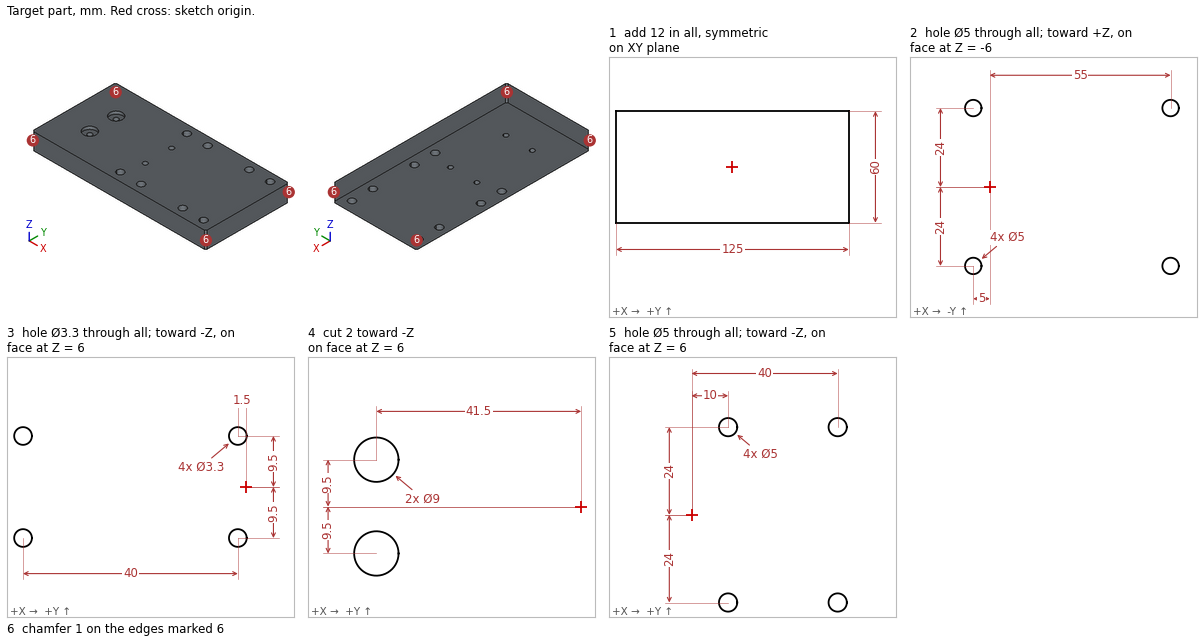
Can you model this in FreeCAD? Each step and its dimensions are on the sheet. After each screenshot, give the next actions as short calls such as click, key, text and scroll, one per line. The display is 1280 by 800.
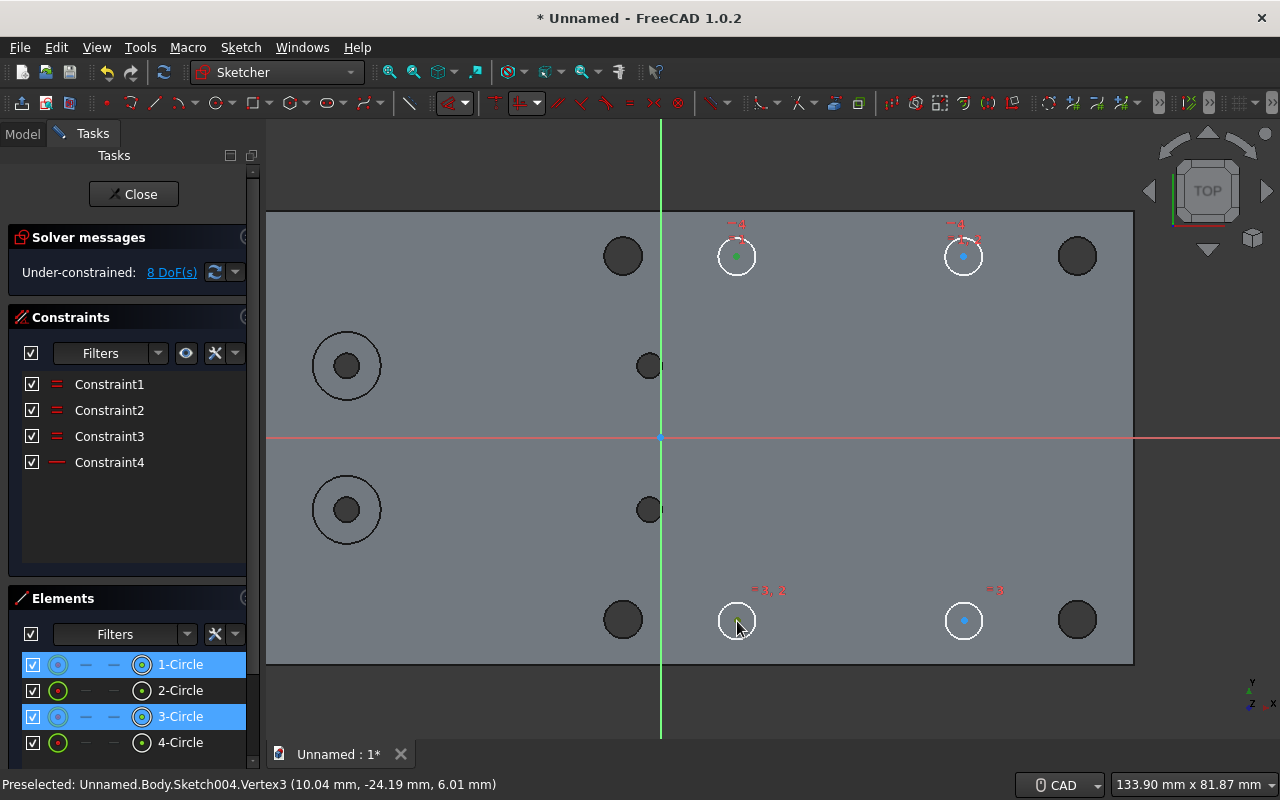
key(v)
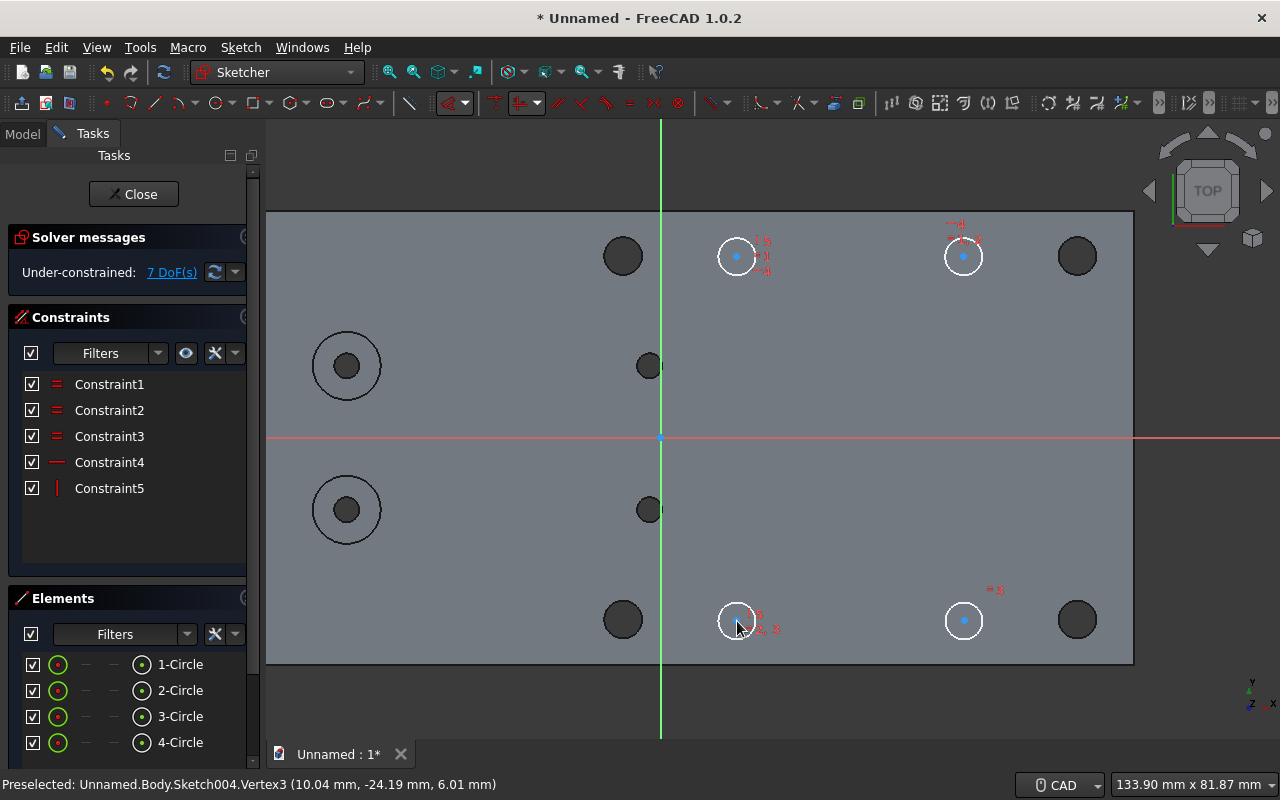
click(964, 257)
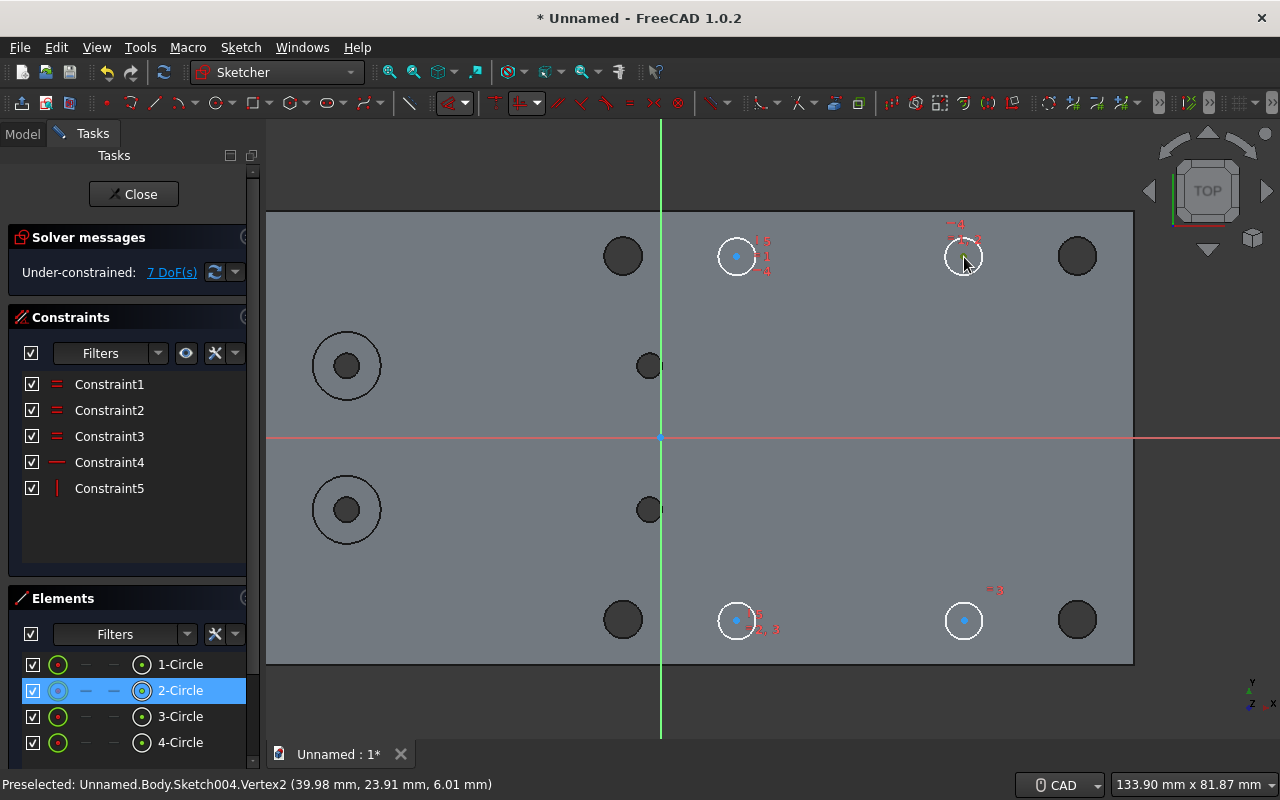
click(964, 621)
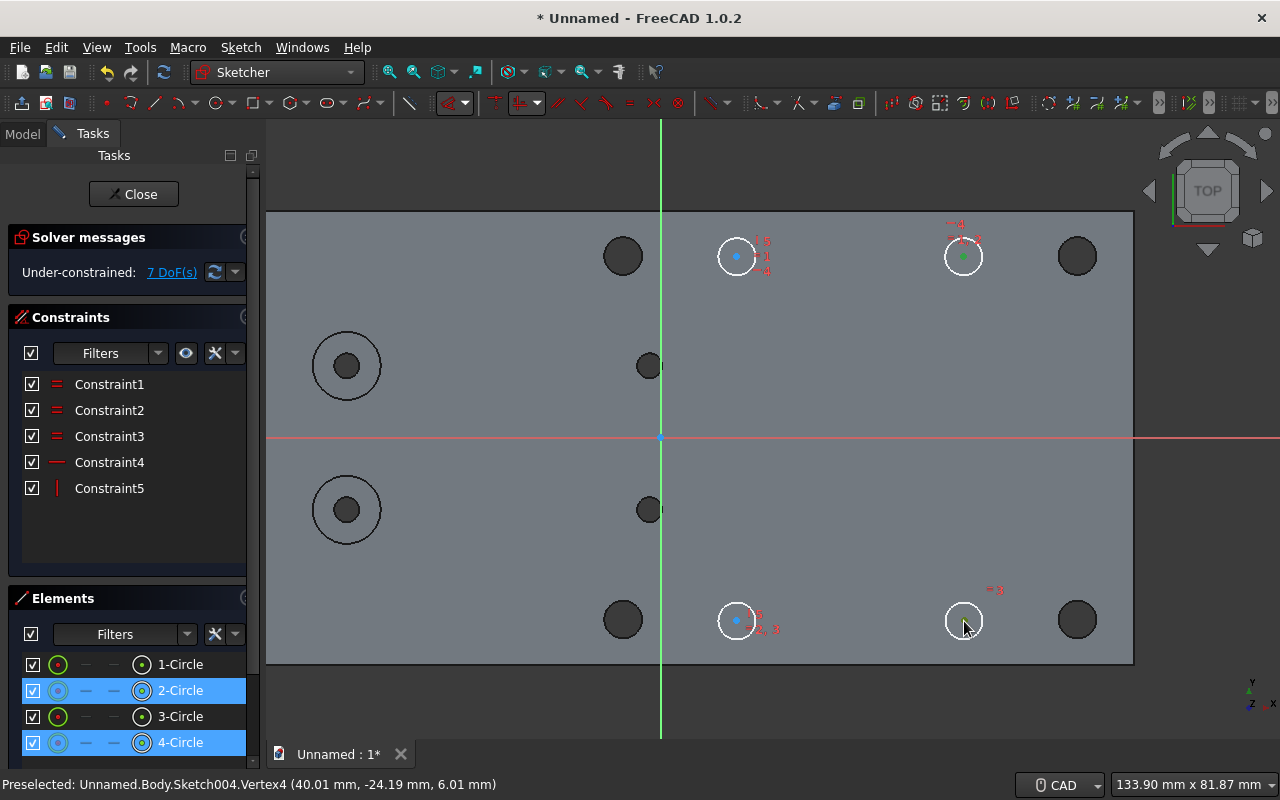
click(540, 104)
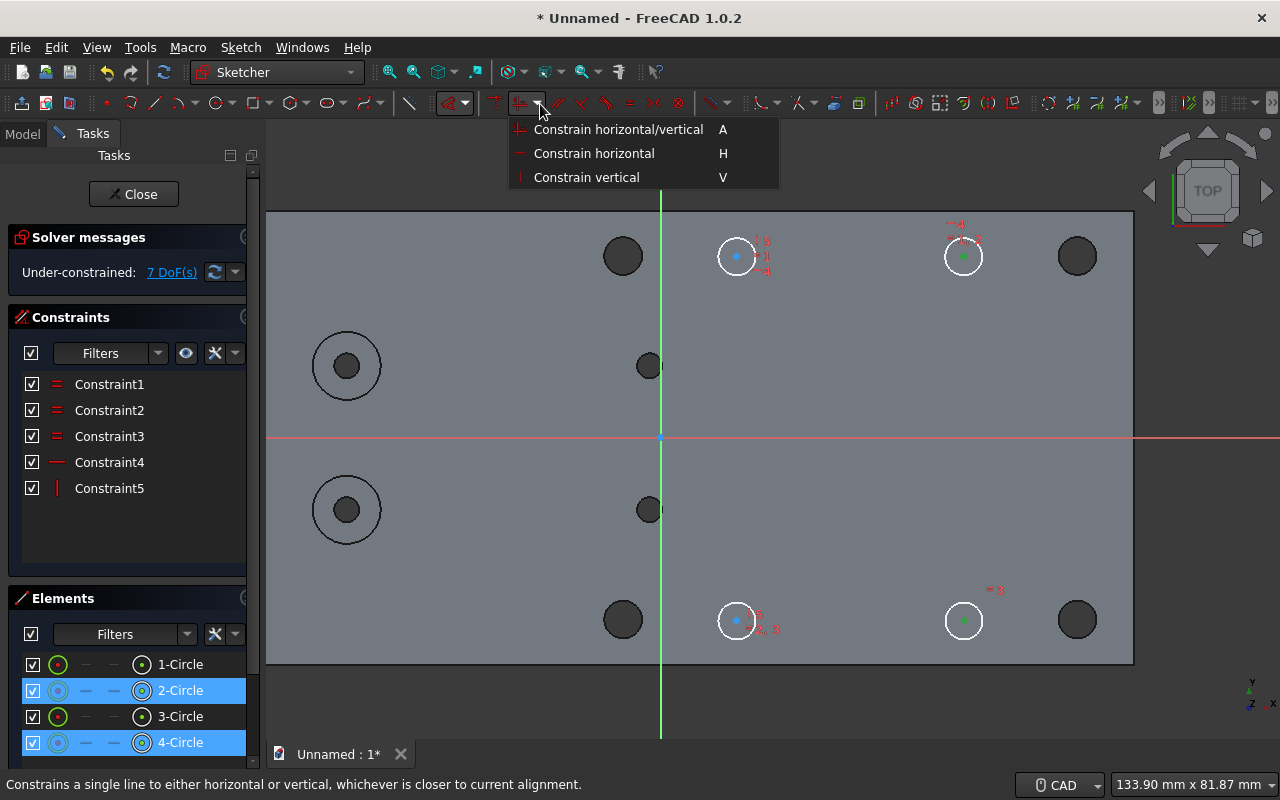
click(644, 177)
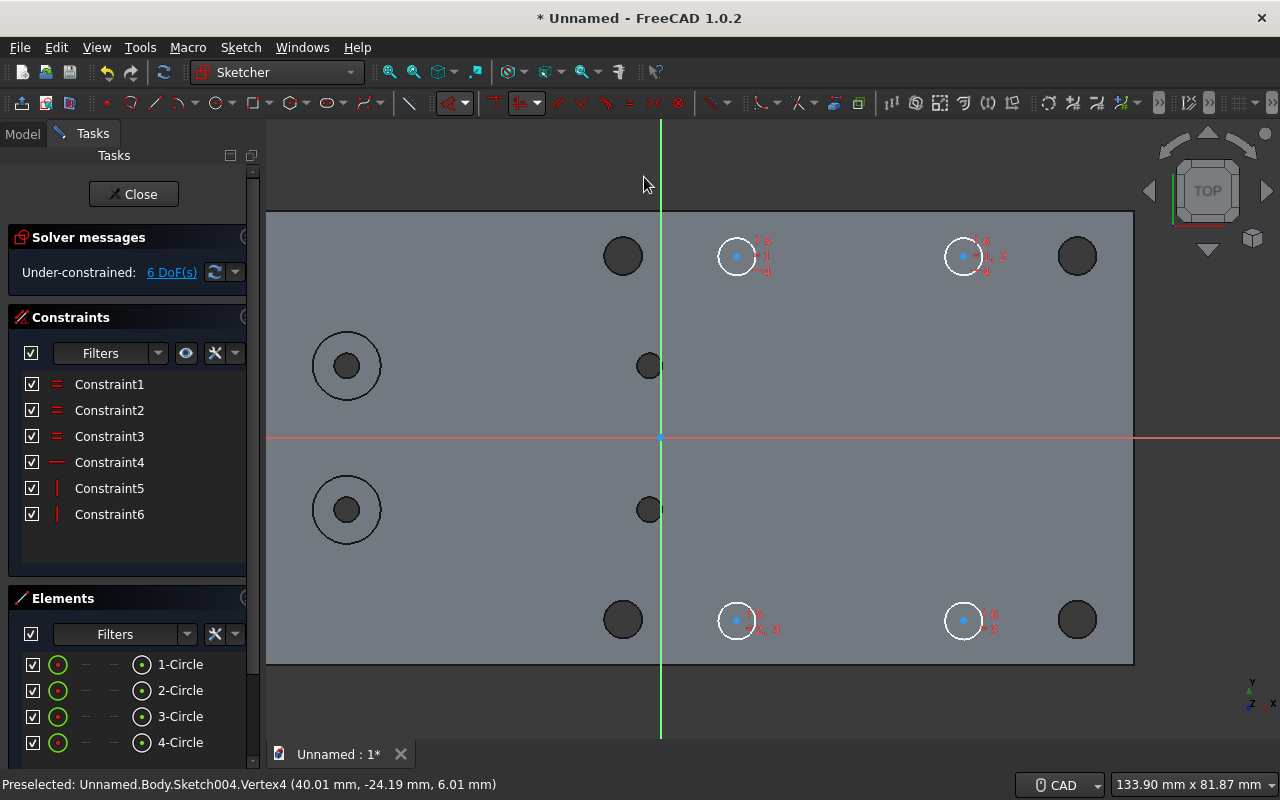
click(737, 621)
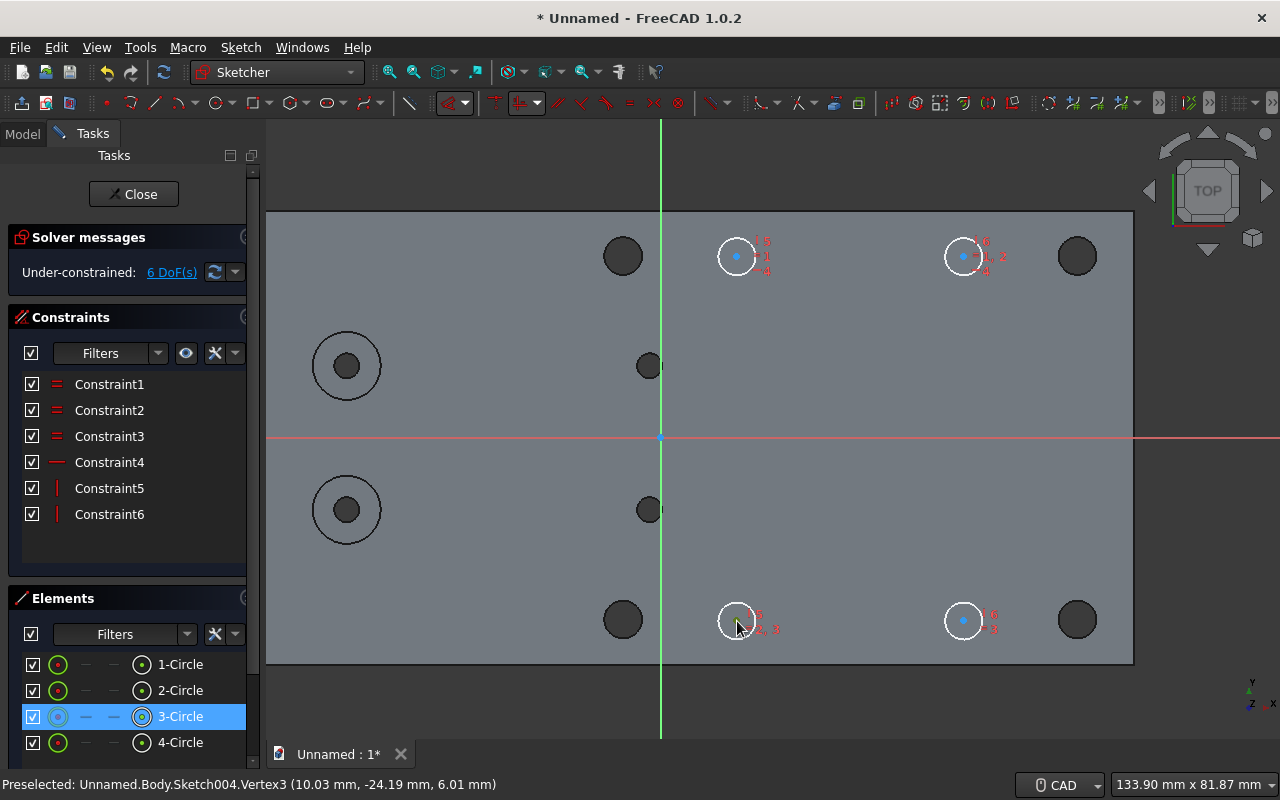
click(964, 621)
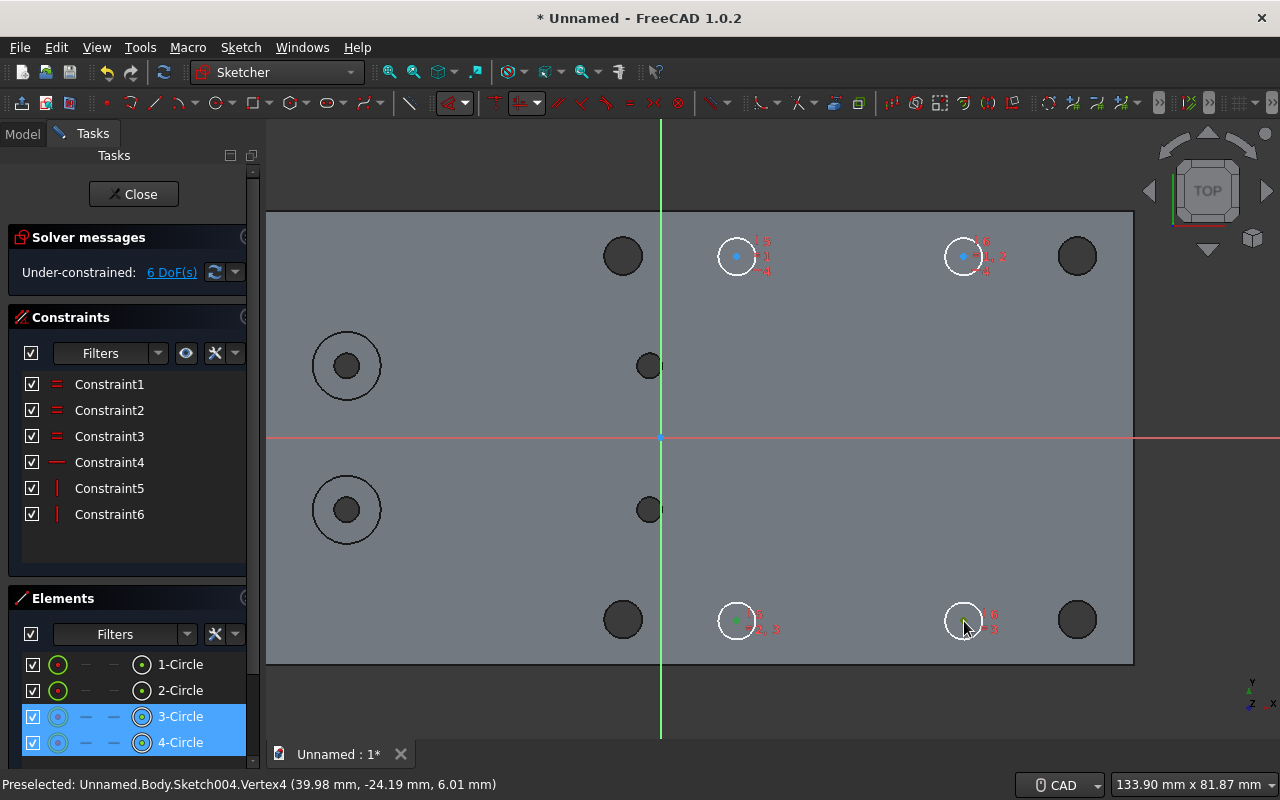
key(h)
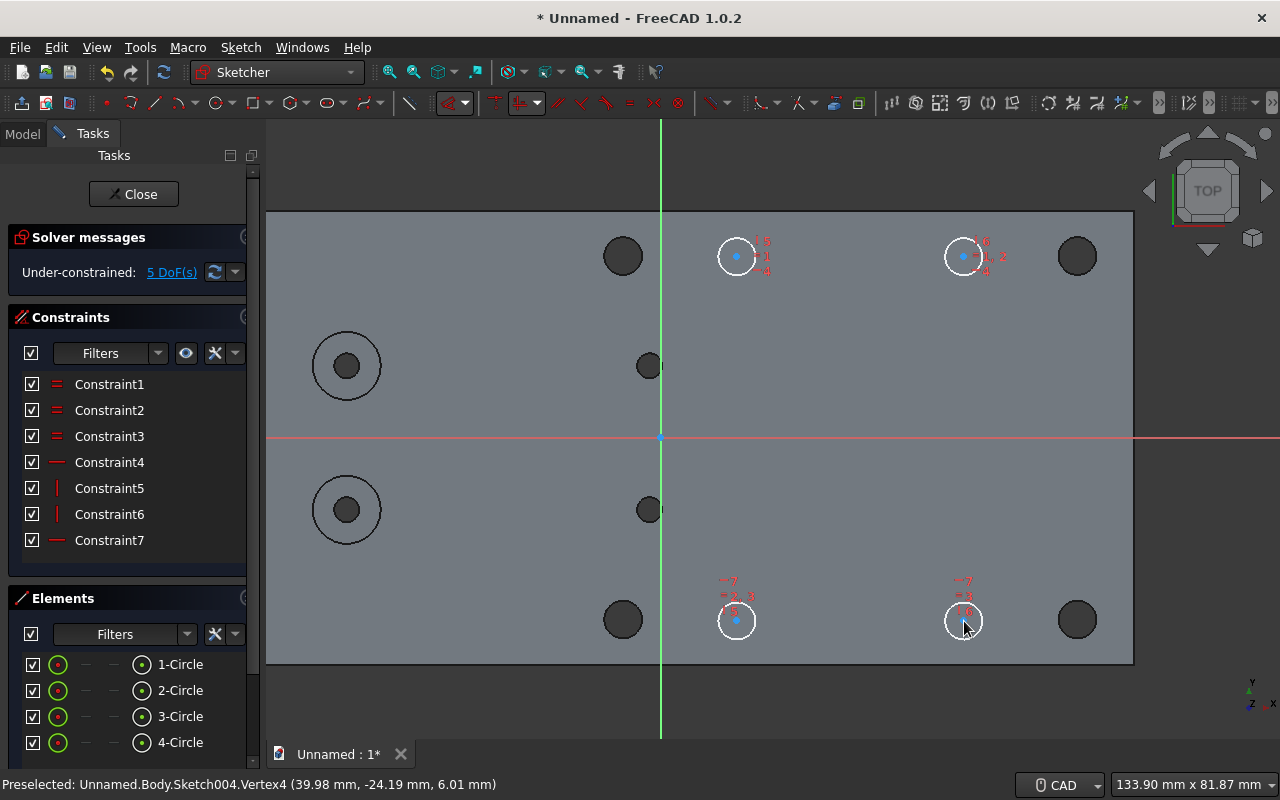
click(750, 244)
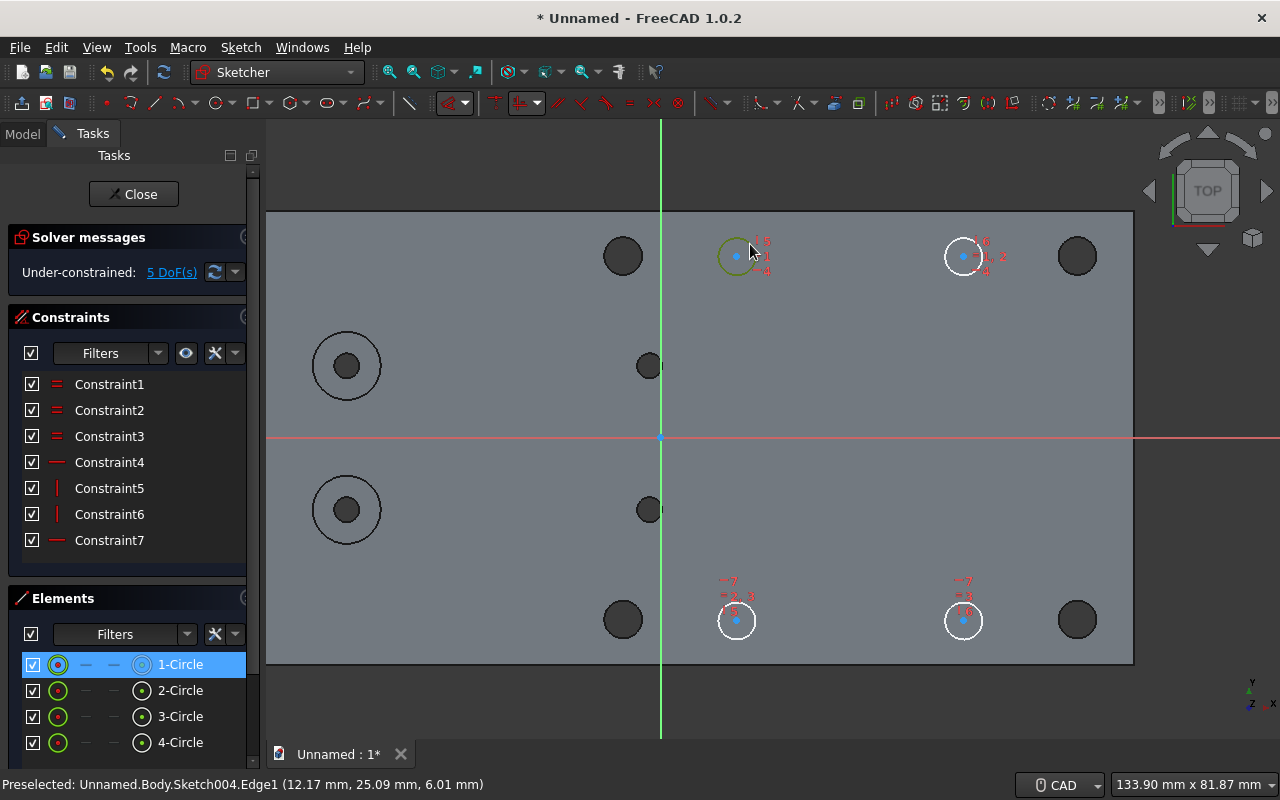
key(k)
key(o)